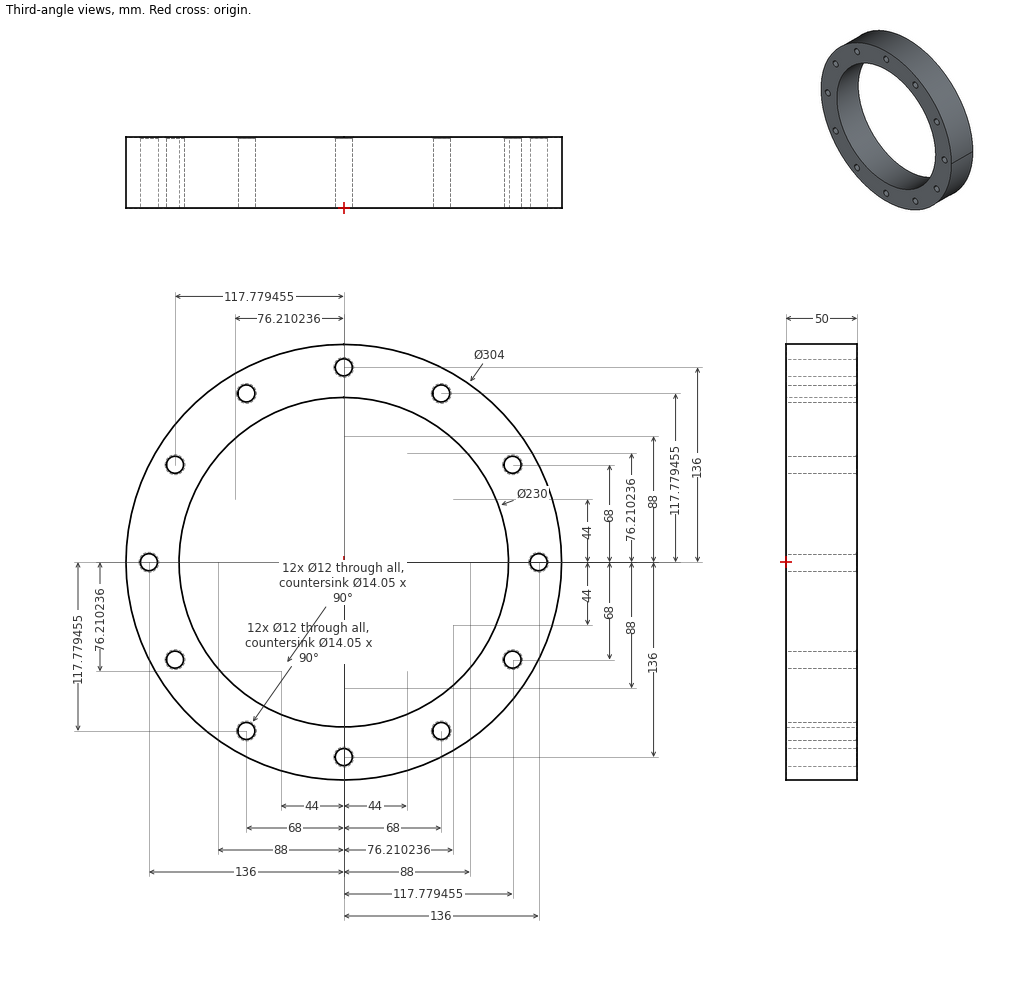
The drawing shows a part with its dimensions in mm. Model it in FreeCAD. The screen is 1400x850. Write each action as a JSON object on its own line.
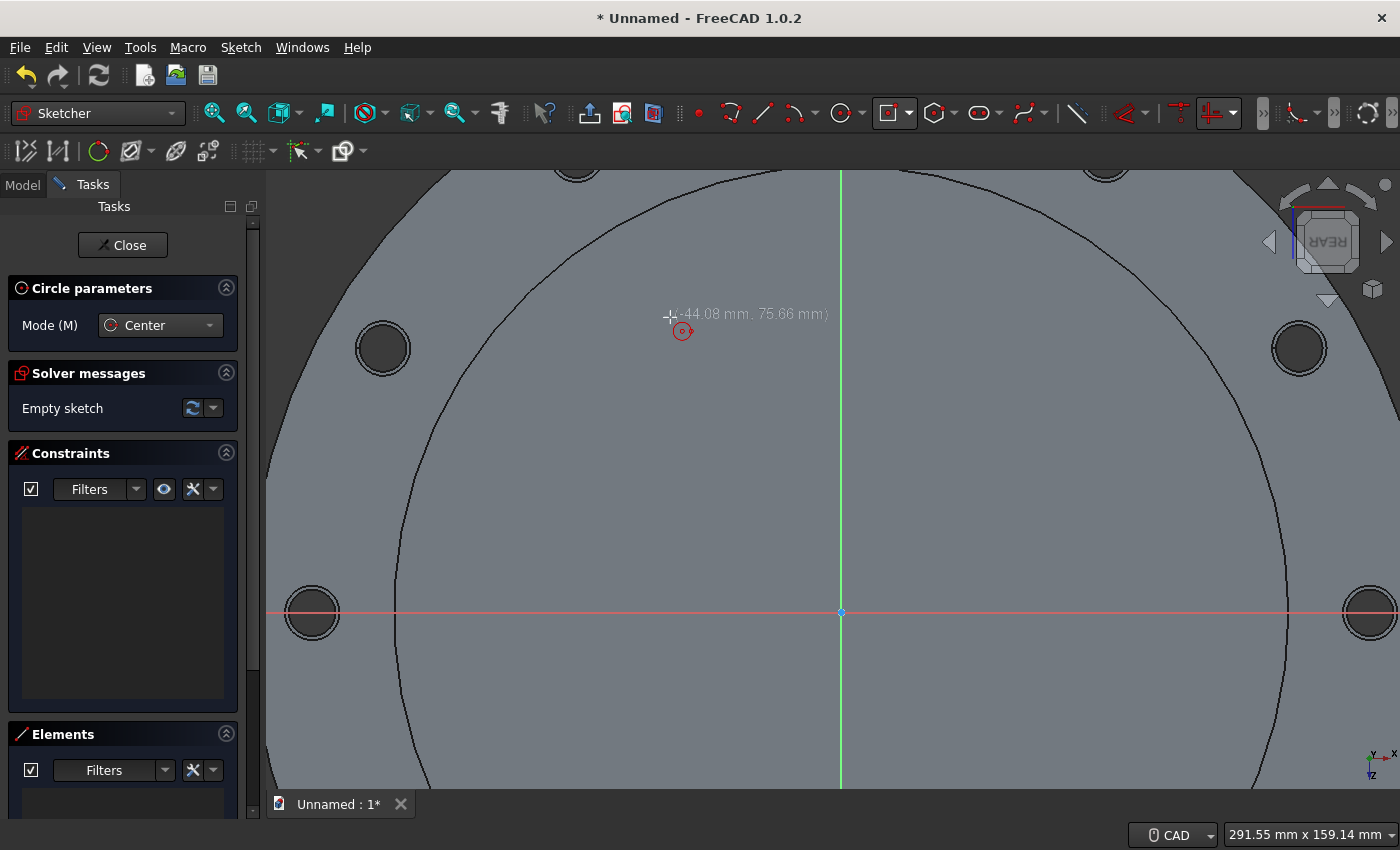
{"action": "left_click", "coordinate": [670, 316]}
{"action": "left_click", "coordinate": [687, 300]}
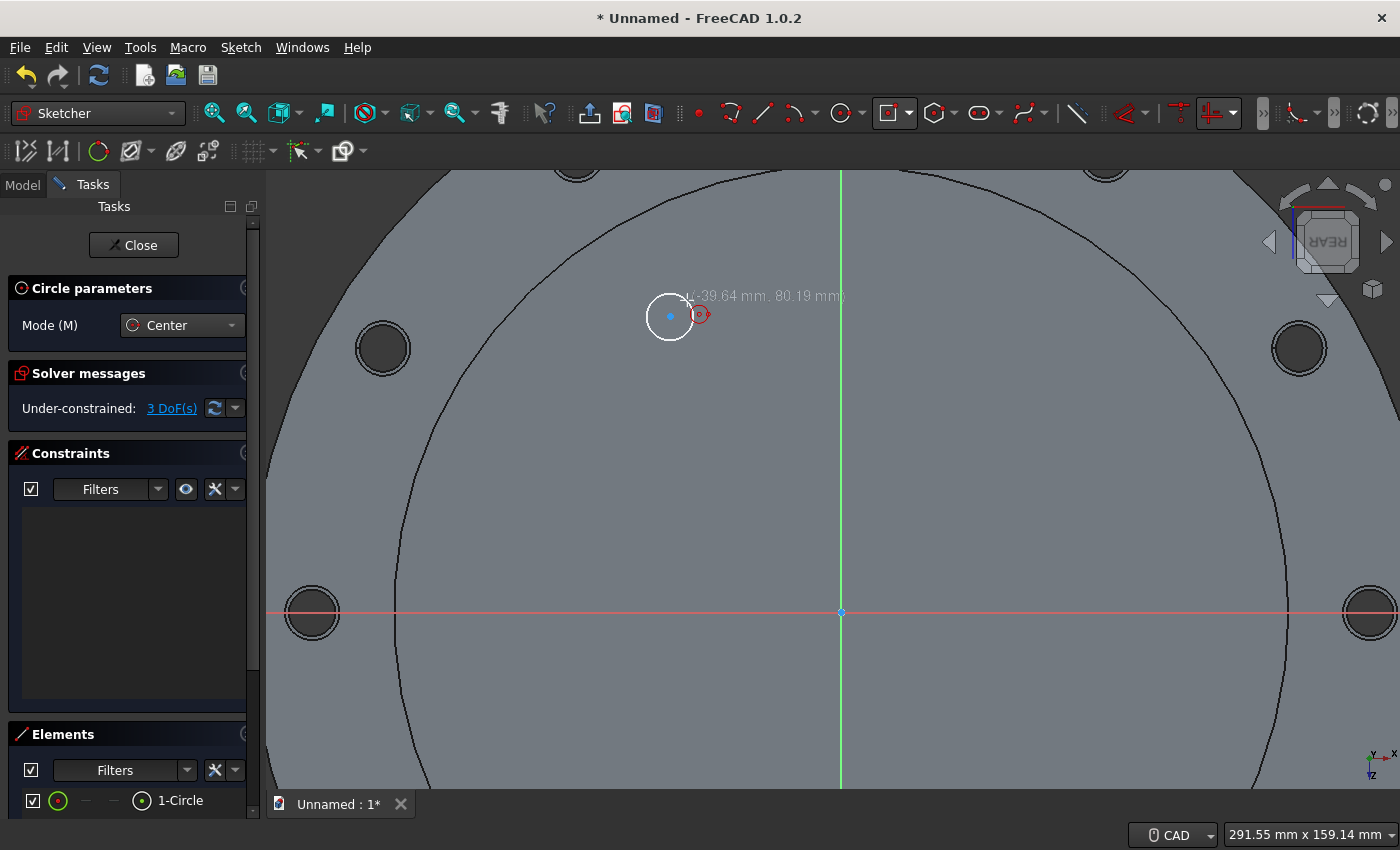
{"action": "left_click", "coordinate": [841, 271]}
{"action": "left_click", "coordinate": [858, 254]}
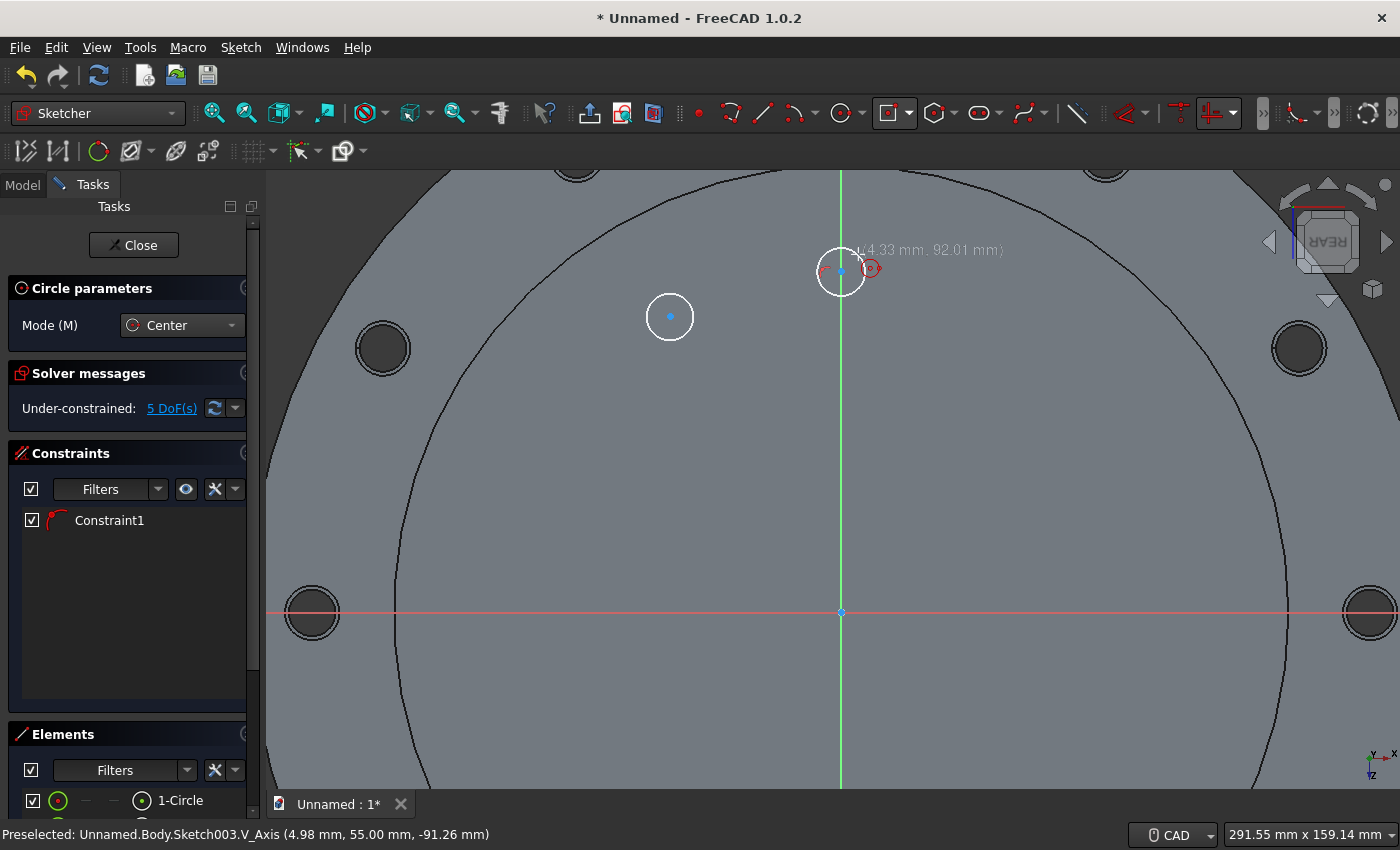
{"action": "left_click", "coordinate": [1012, 316]}
{"action": "left_click", "coordinate": [1029, 300]}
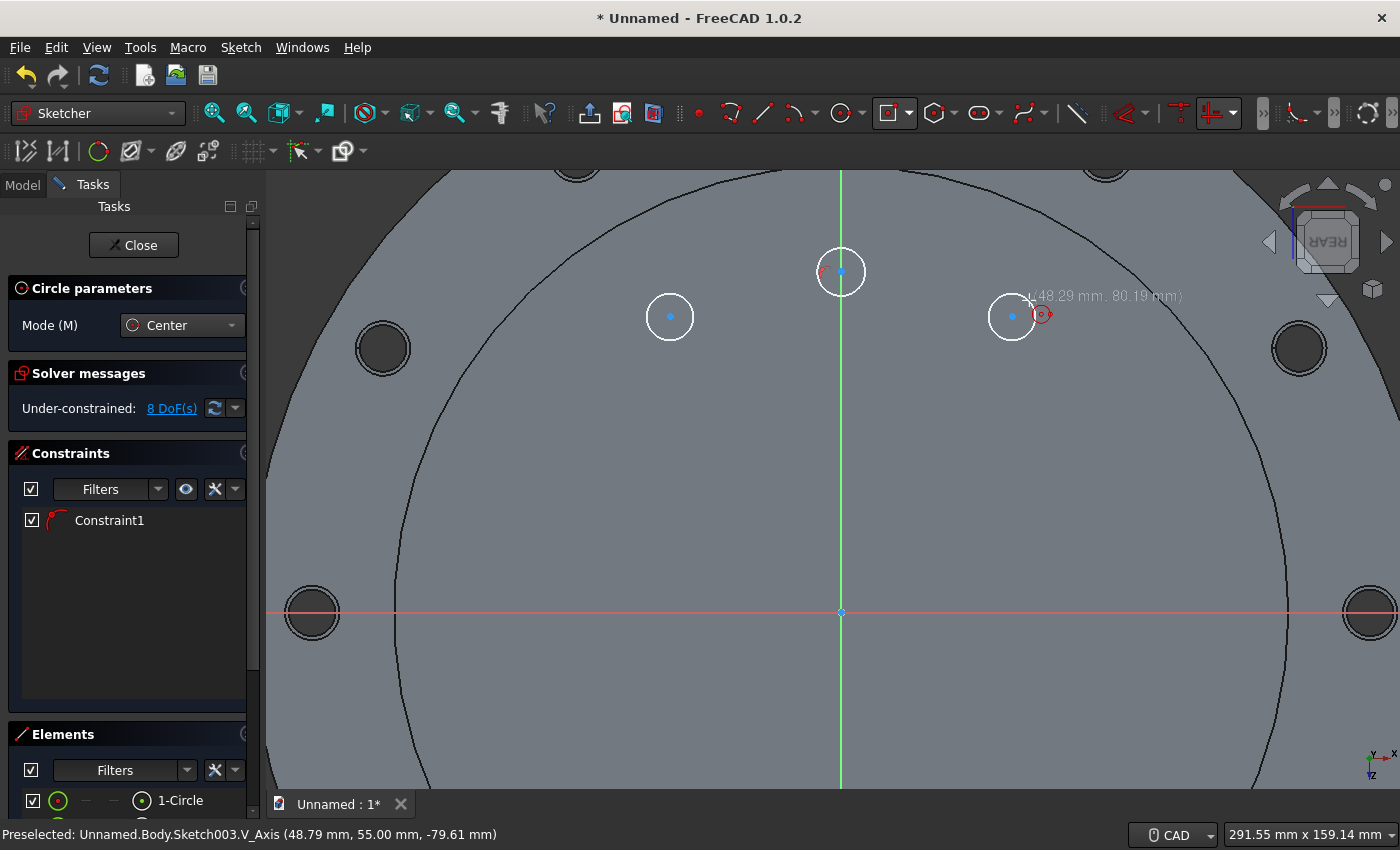
{"action": "left_click", "coordinate": [1138, 442]}
{"action": "left_click", "coordinate": [1154, 425]}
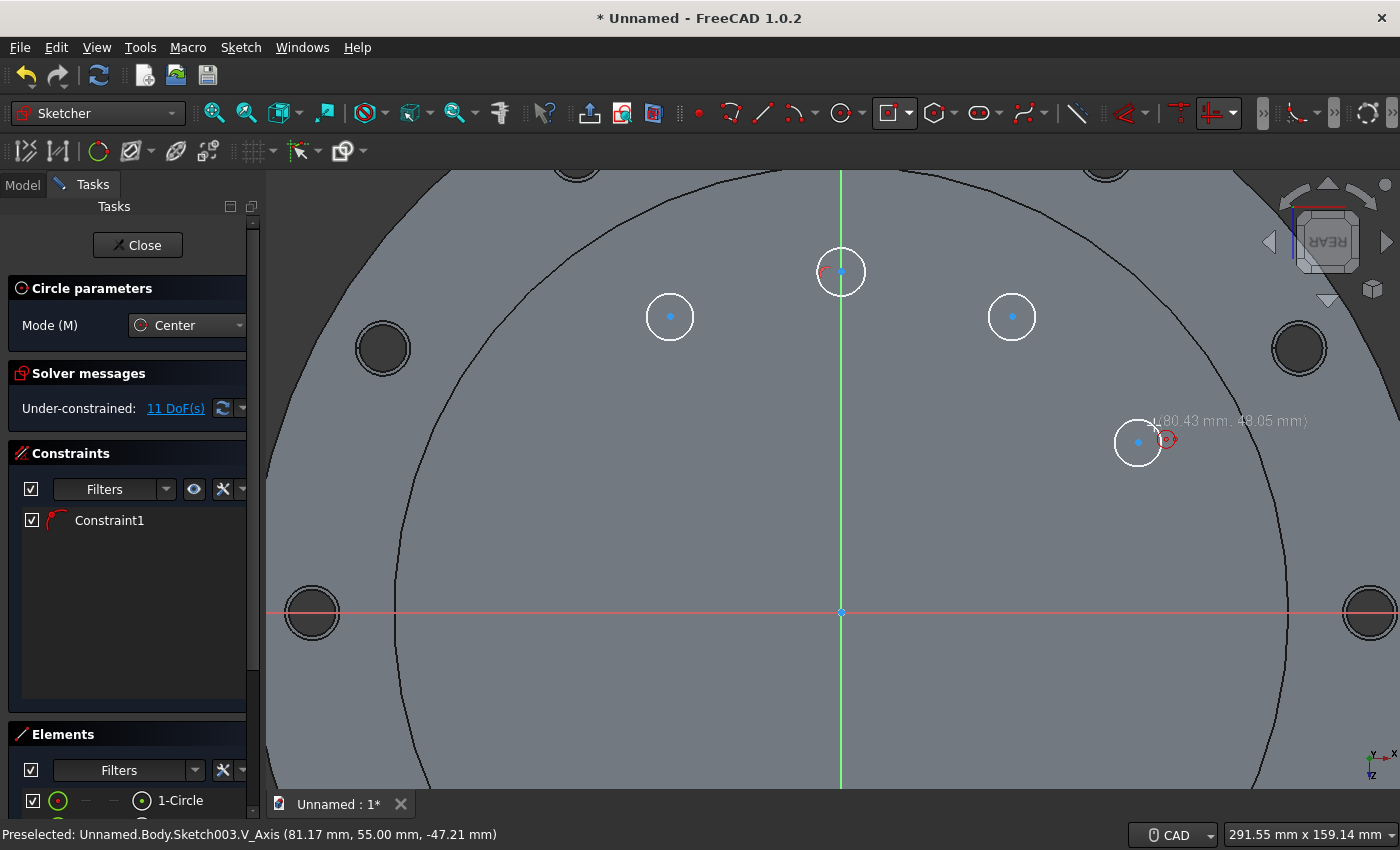
{"action": "left_click", "coordinate": [1183, 613]}
{"action": "left_click", "coordinate": [1200, 596]}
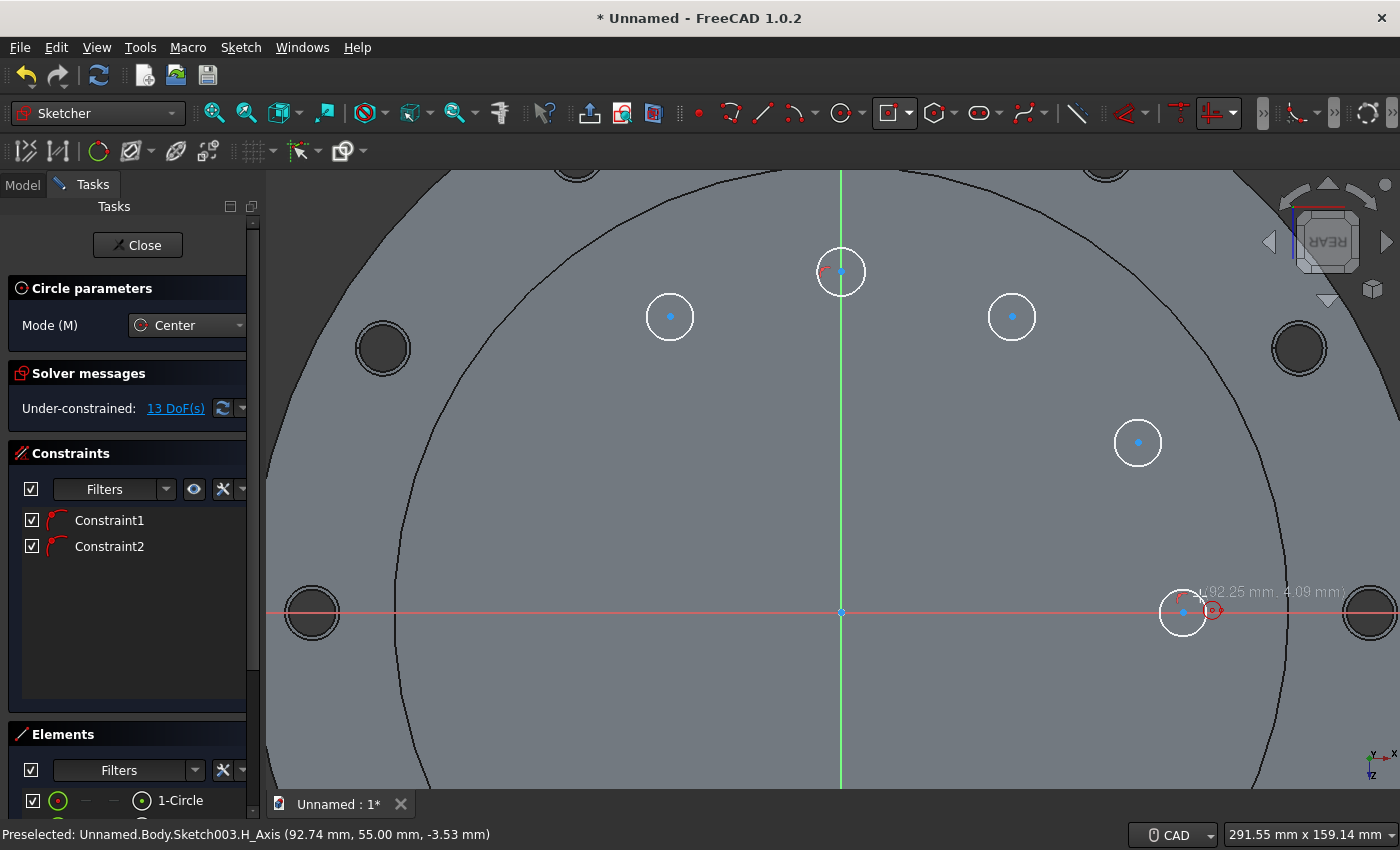
{"action": "scroll", "coordinate": [671, 317], "scroll_direction": "down", "scroll_amount": 3}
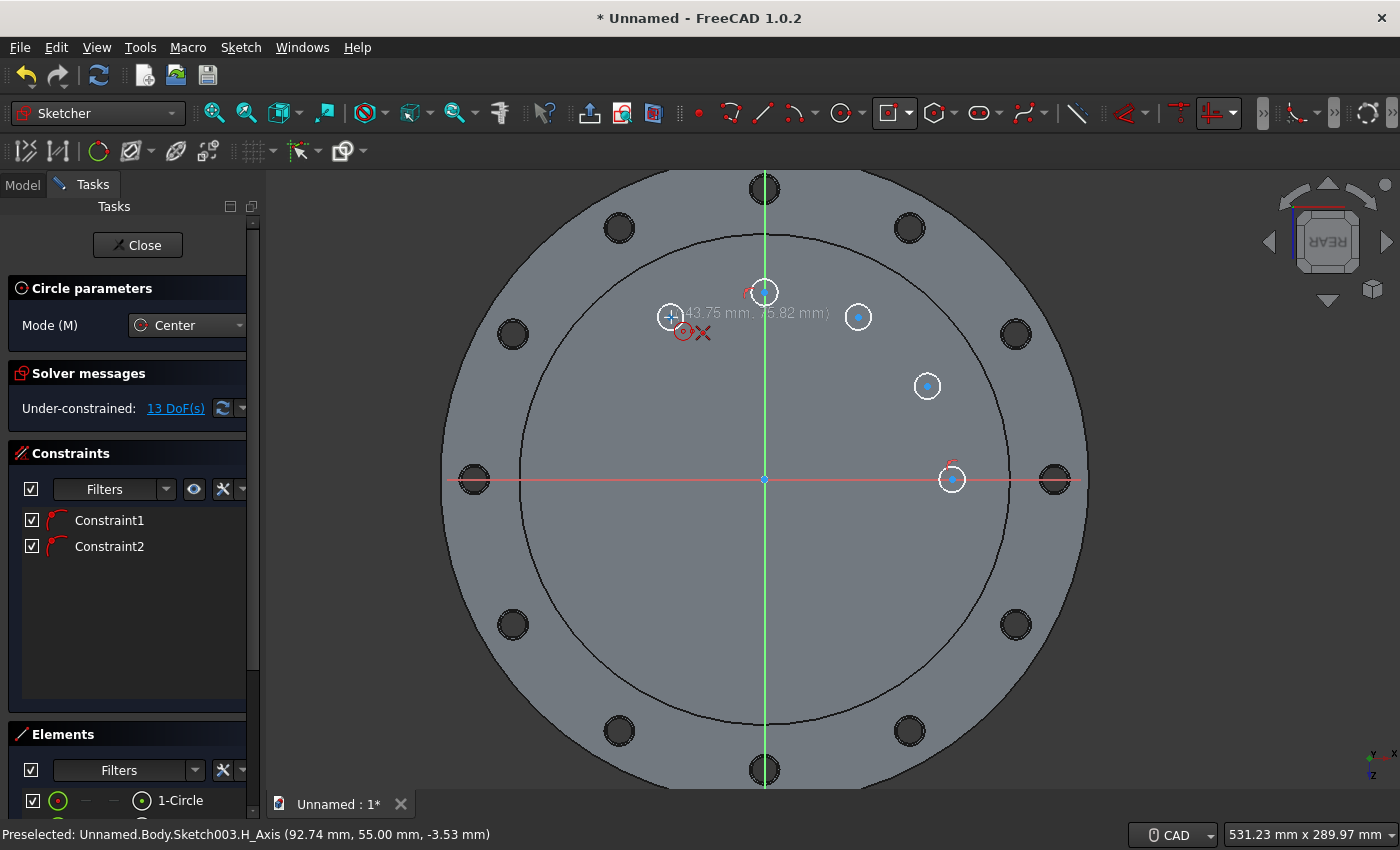
{"action": "scroll", "coordinate": [927, 573], "scroll_direction": "up", "scroll_amount": 3}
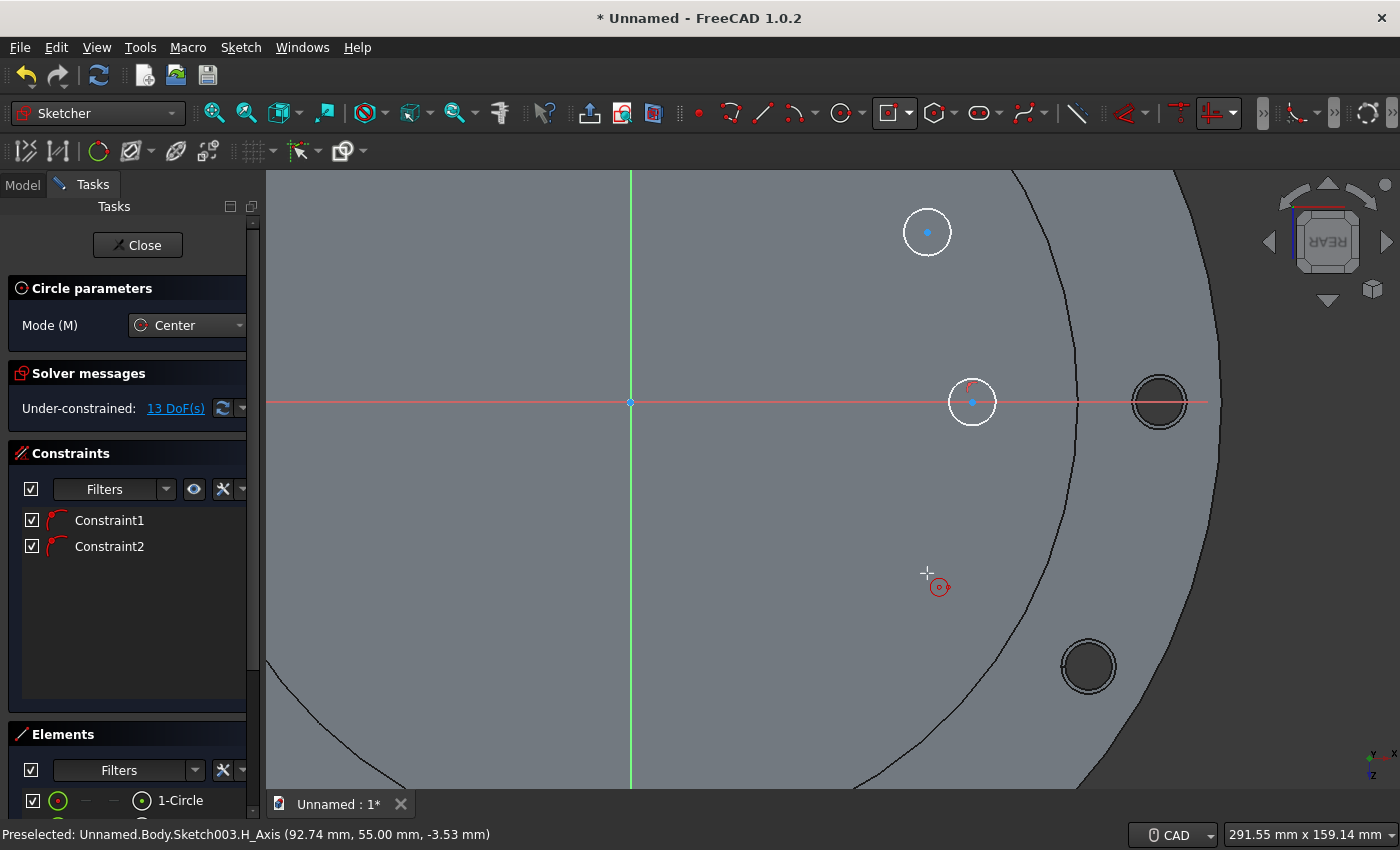
{"action": "left_click", "coordinate": [927, 573]}
{"action": "left_click", "coordinate": [943, 557]}